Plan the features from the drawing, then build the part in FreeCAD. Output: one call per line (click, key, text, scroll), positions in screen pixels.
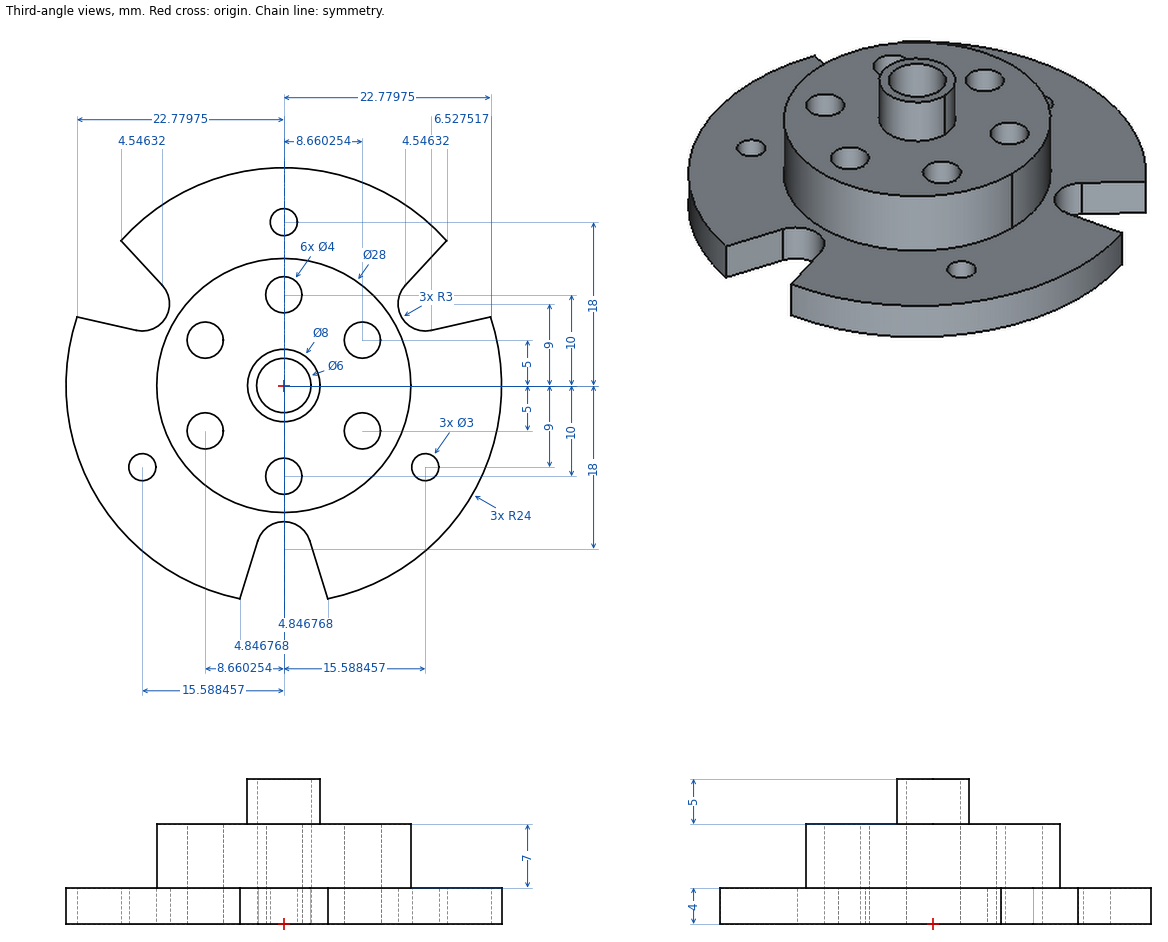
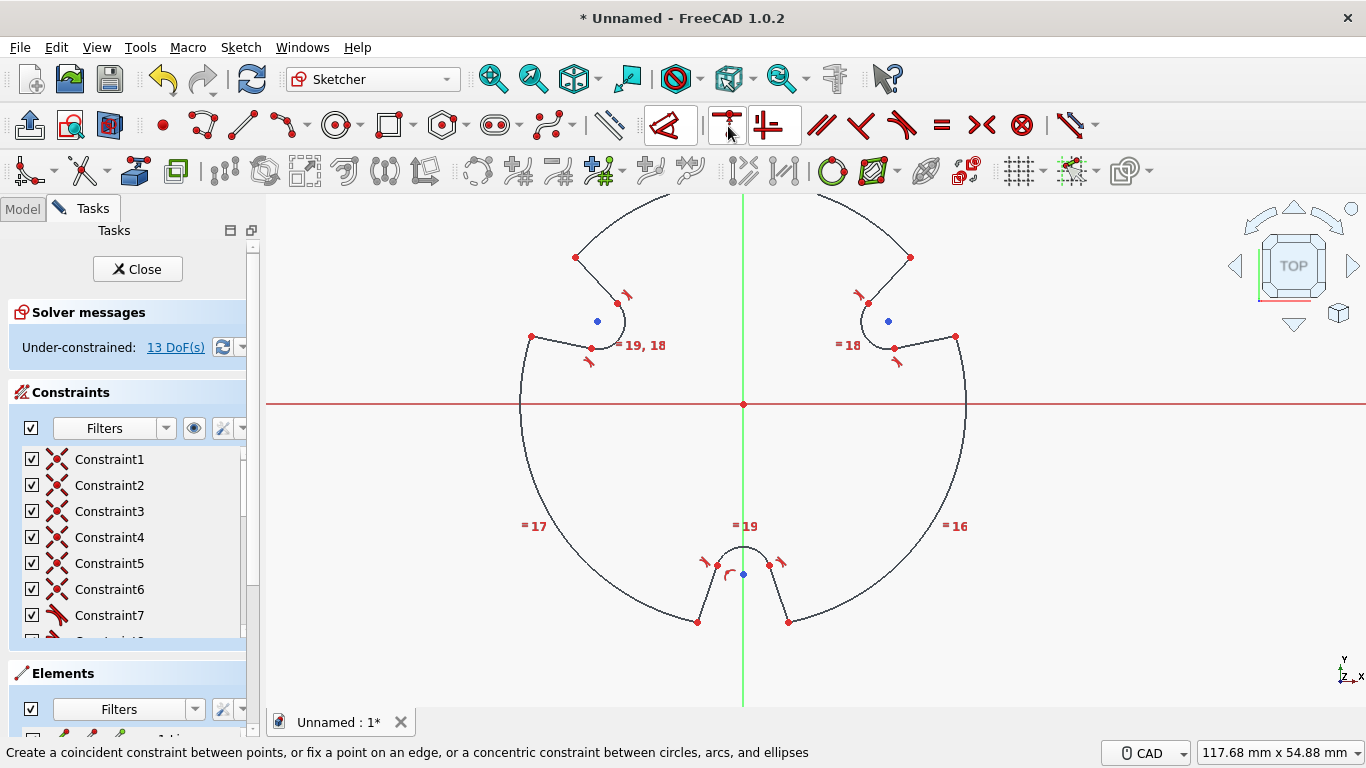
click(889, 322)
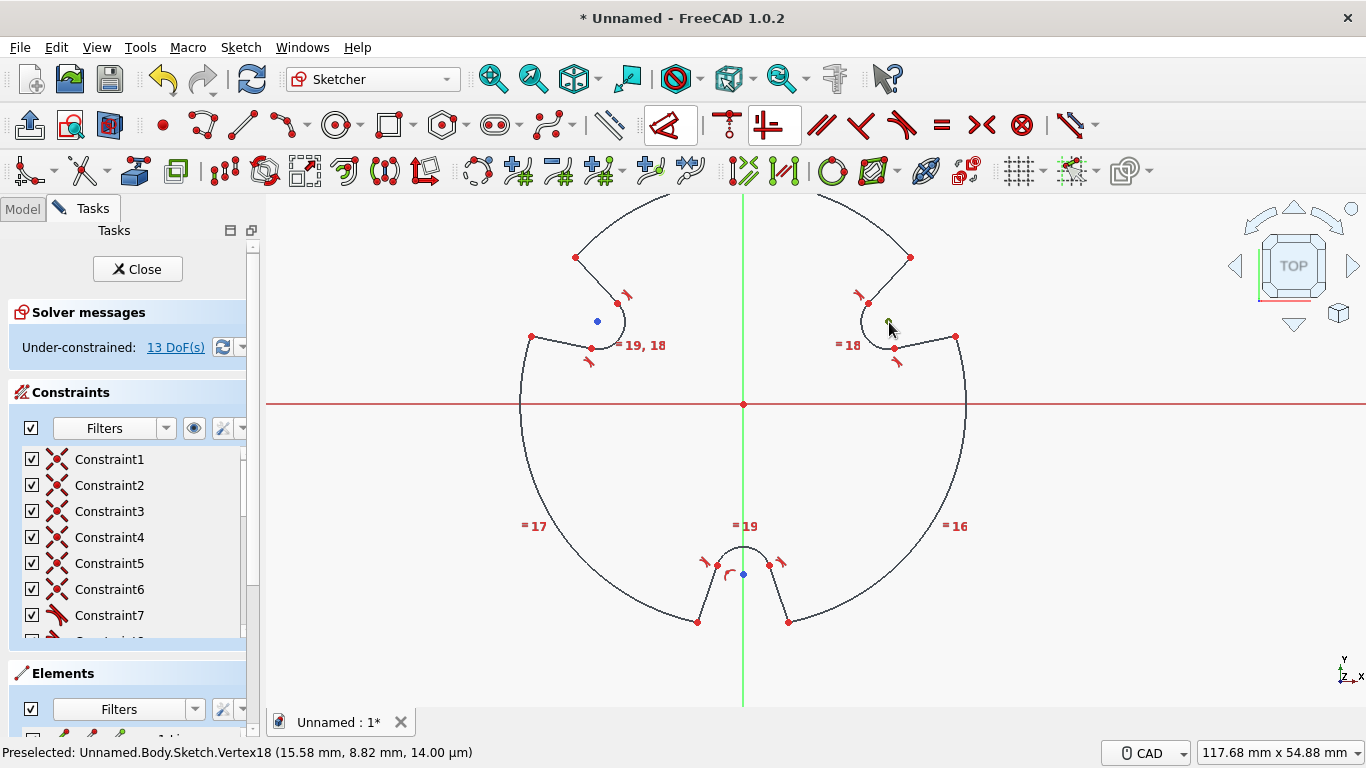
click(598, 322)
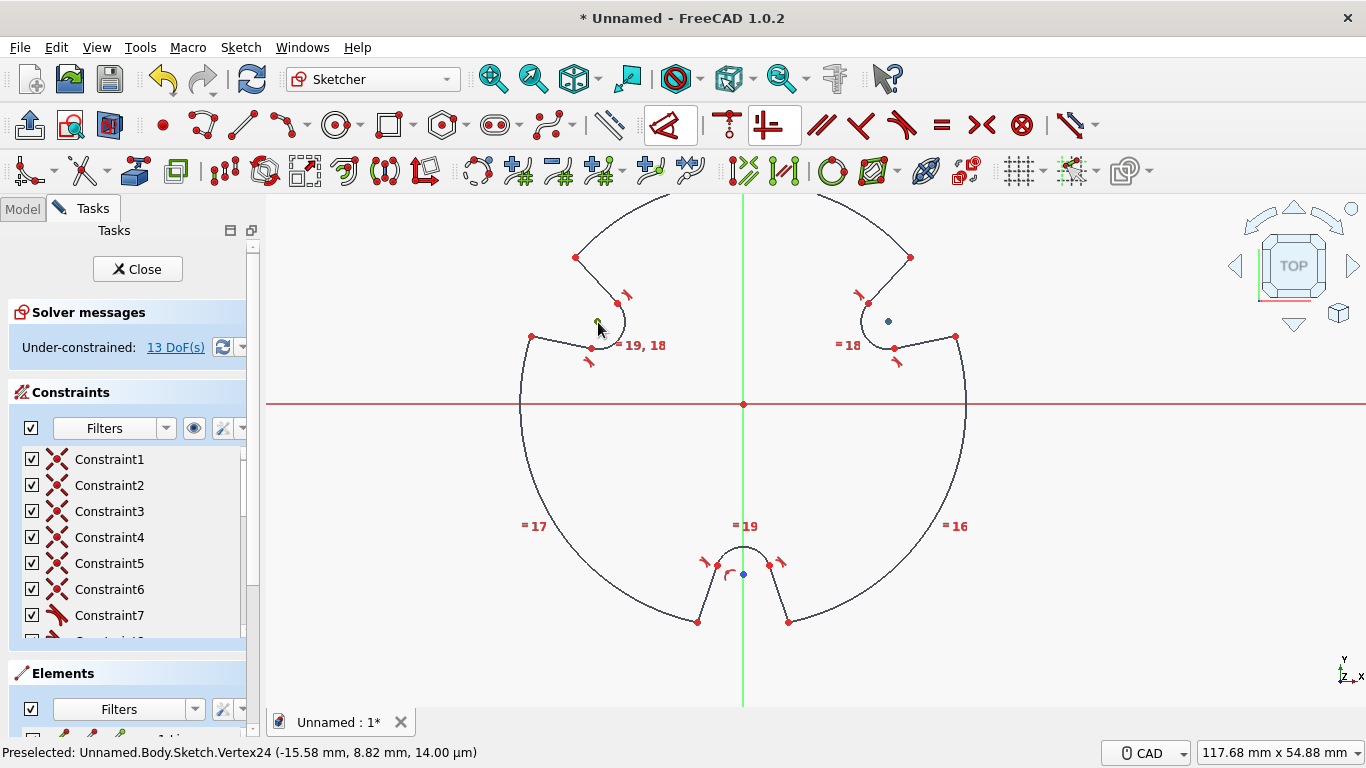
click(743, 646)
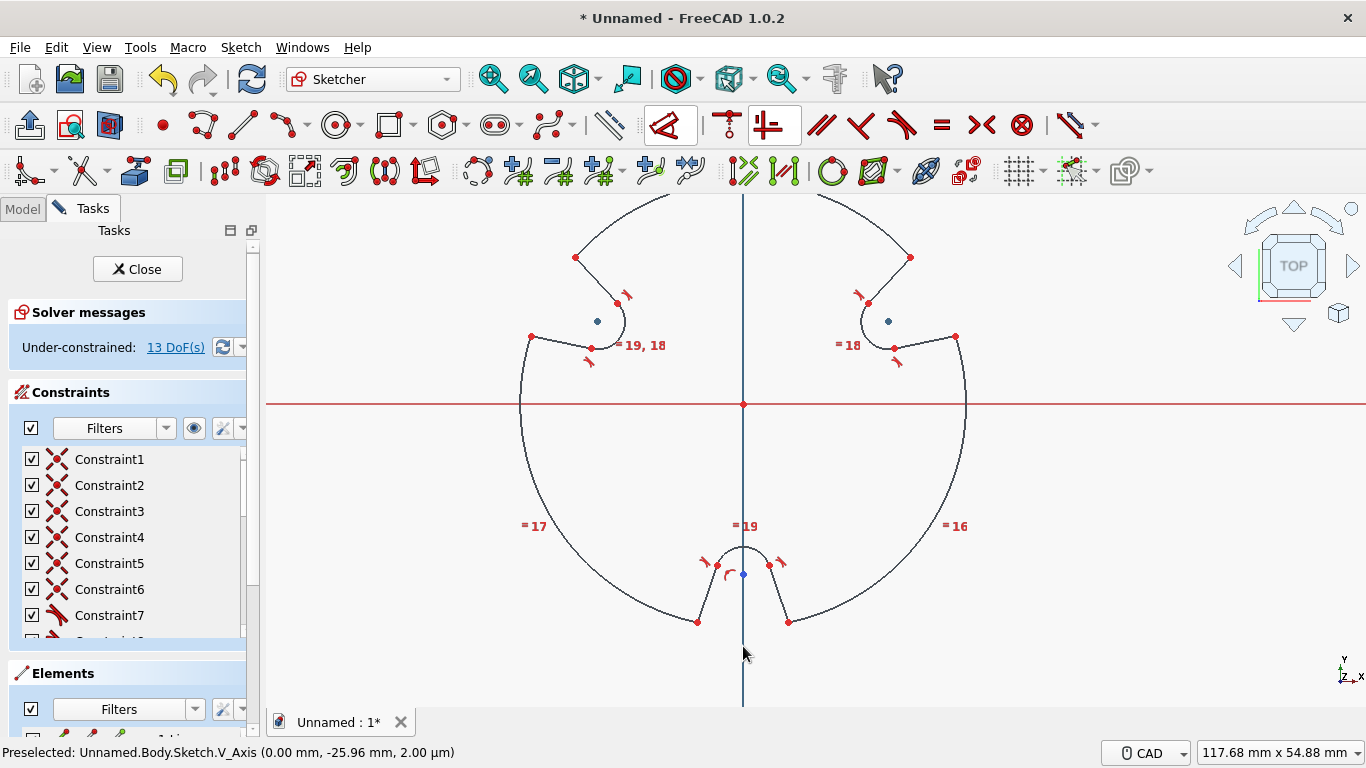
key(s)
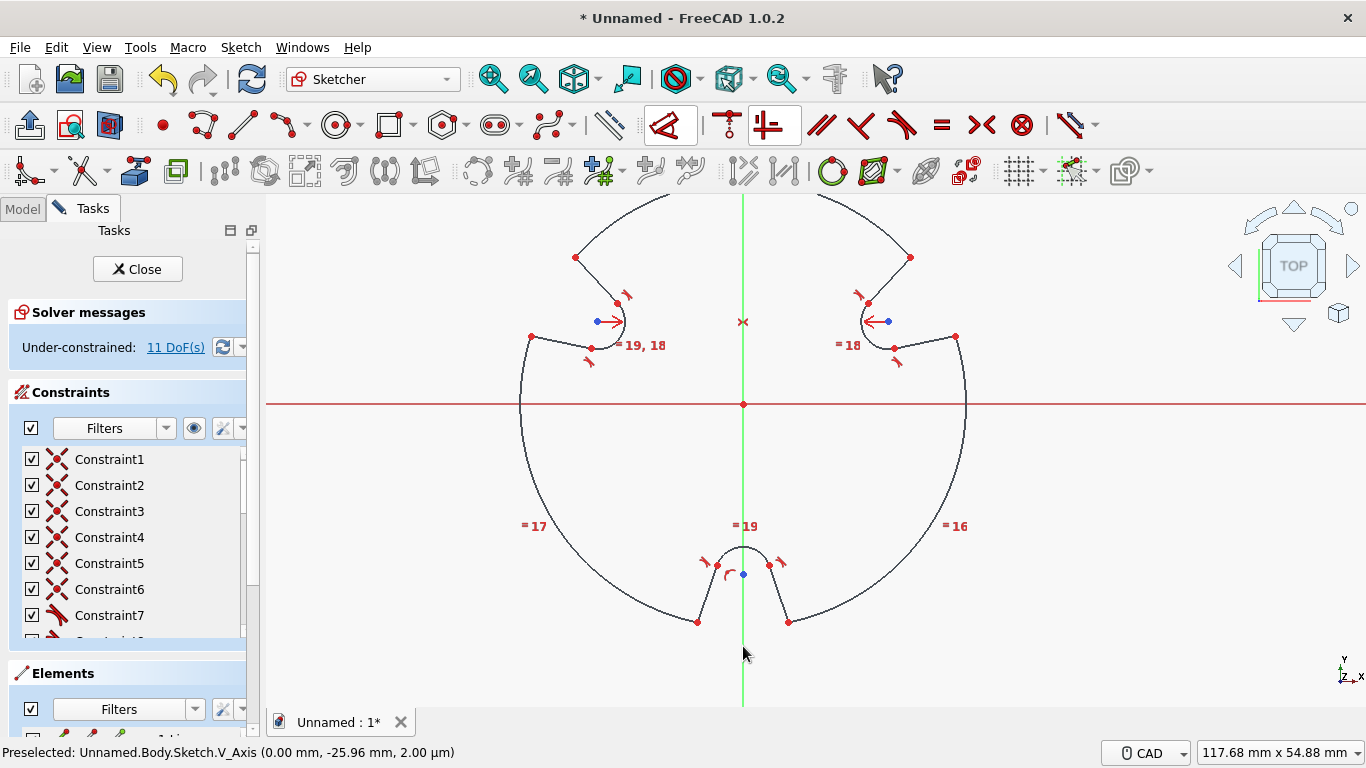
key(d)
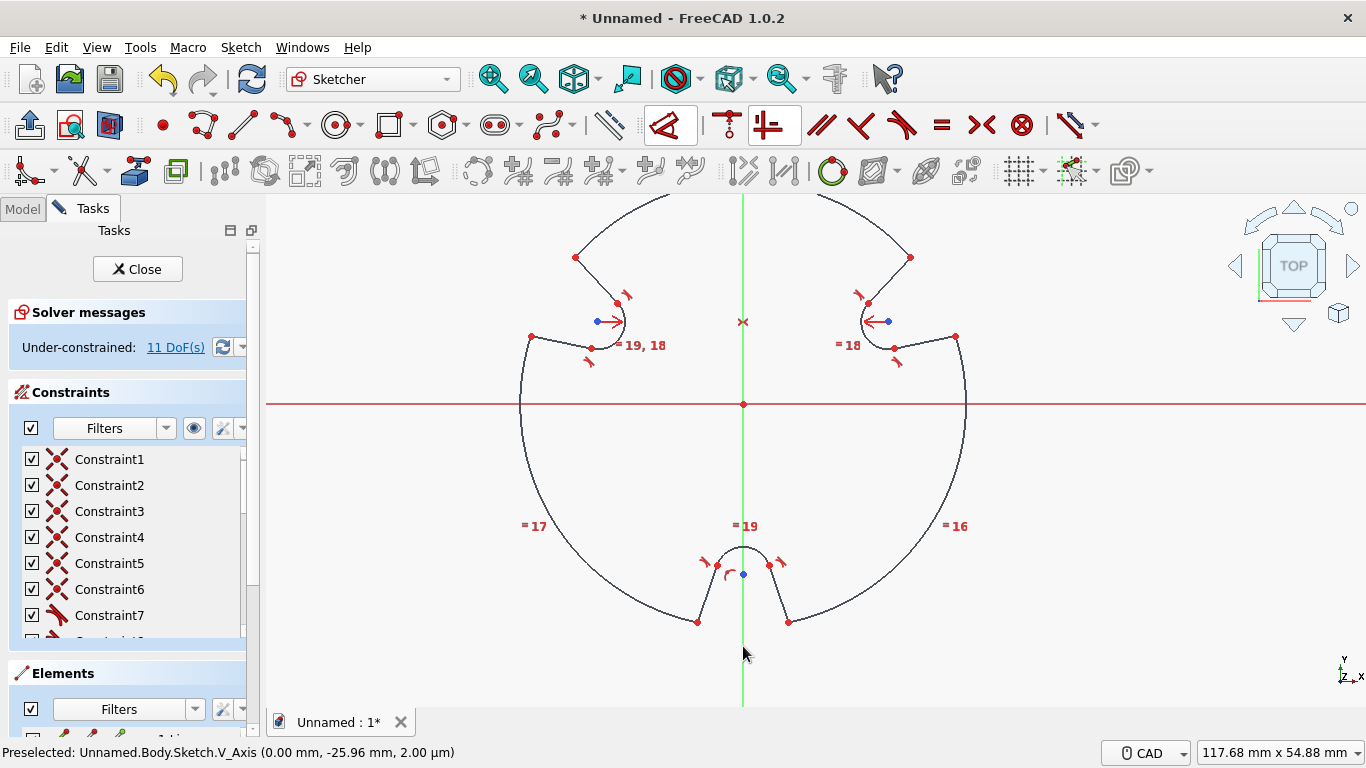
click(888, 574)
click(909, 598)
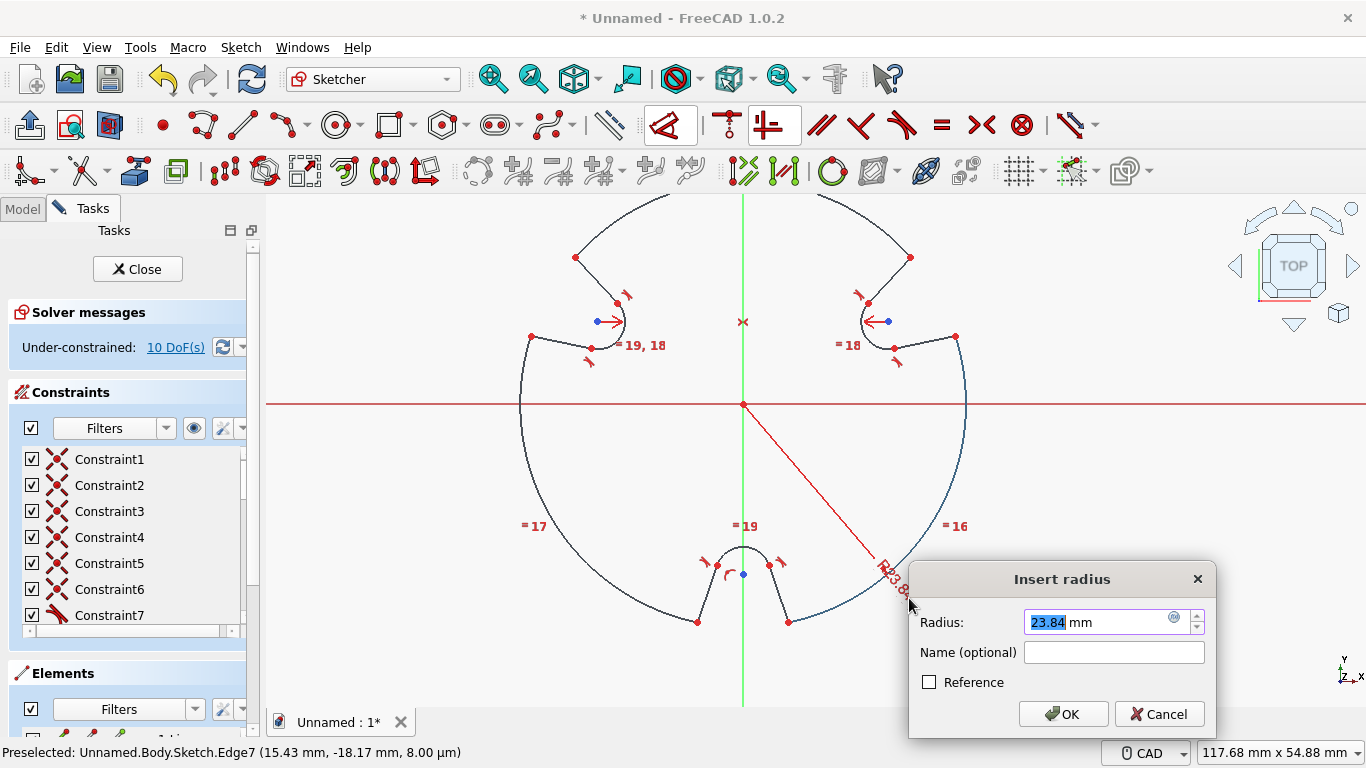
text(24)
key(Return)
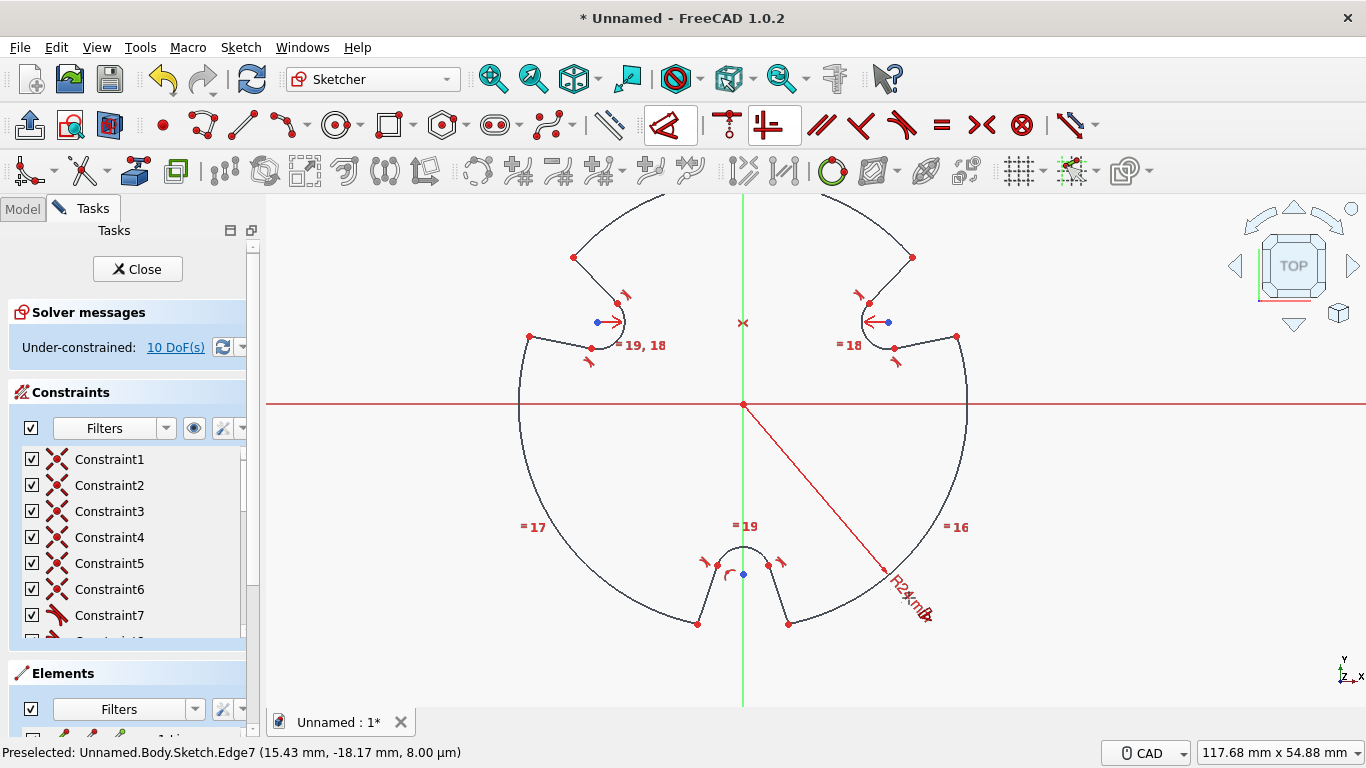
scroll(862, 322, up, 2)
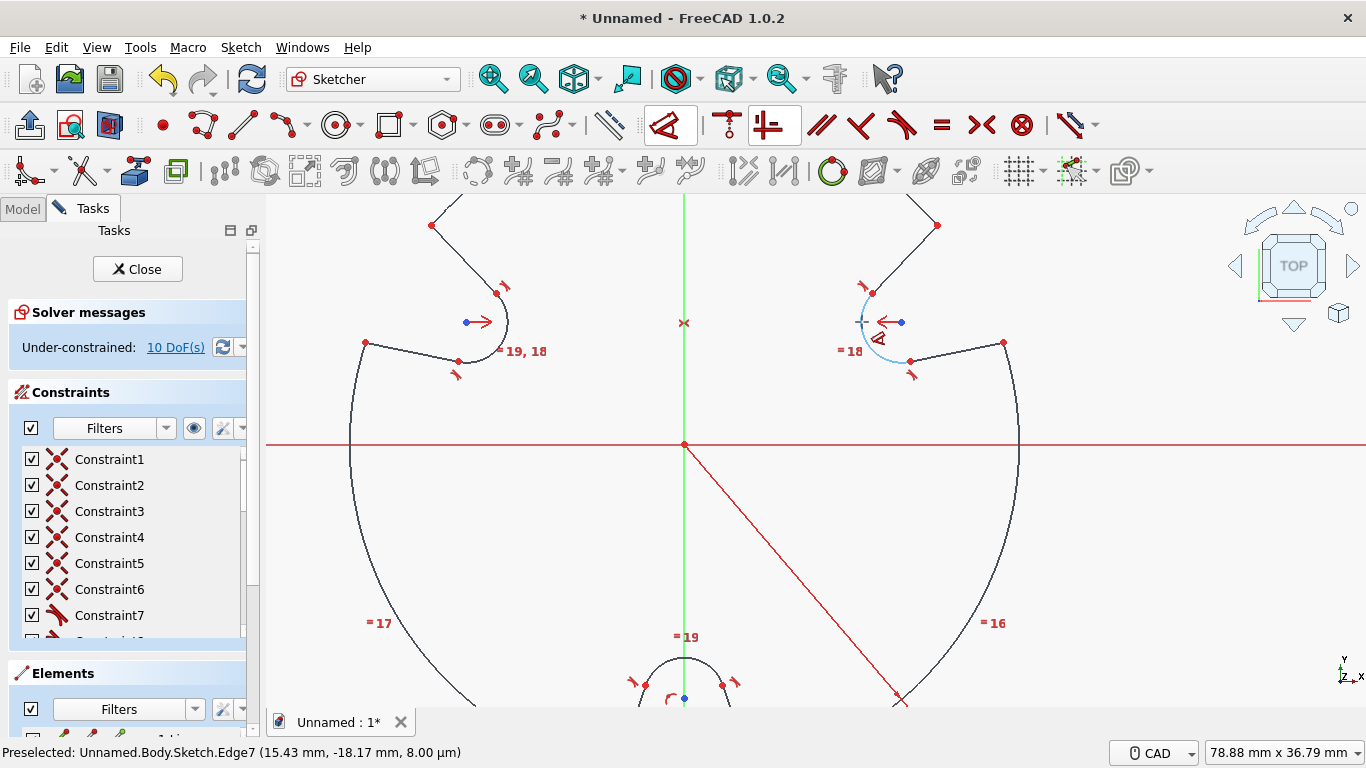
click(861, 322)
click(829, 322)